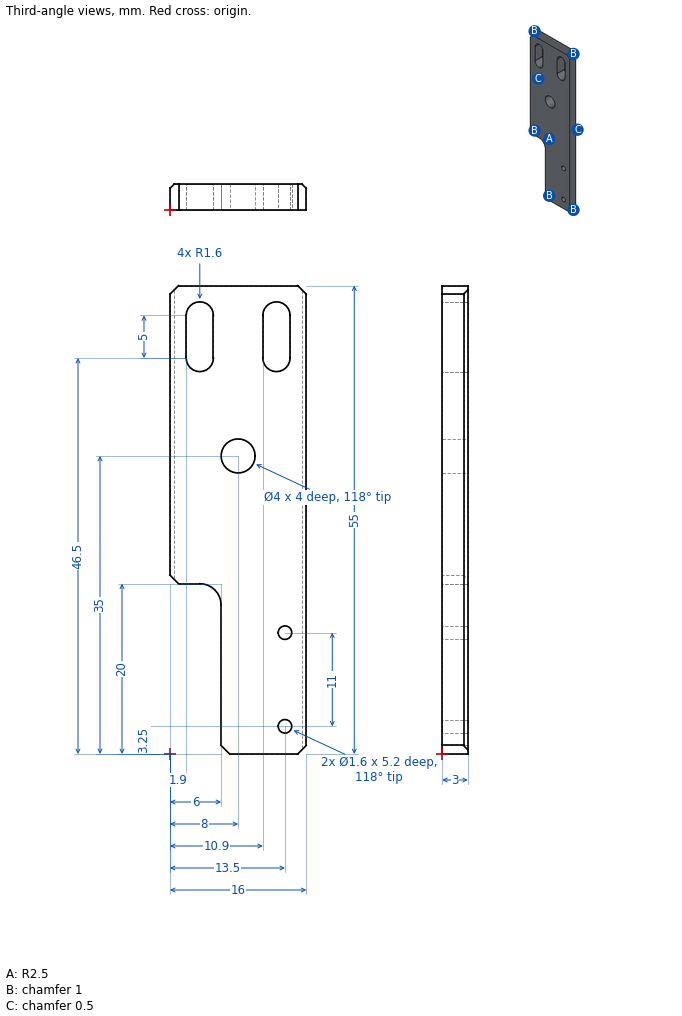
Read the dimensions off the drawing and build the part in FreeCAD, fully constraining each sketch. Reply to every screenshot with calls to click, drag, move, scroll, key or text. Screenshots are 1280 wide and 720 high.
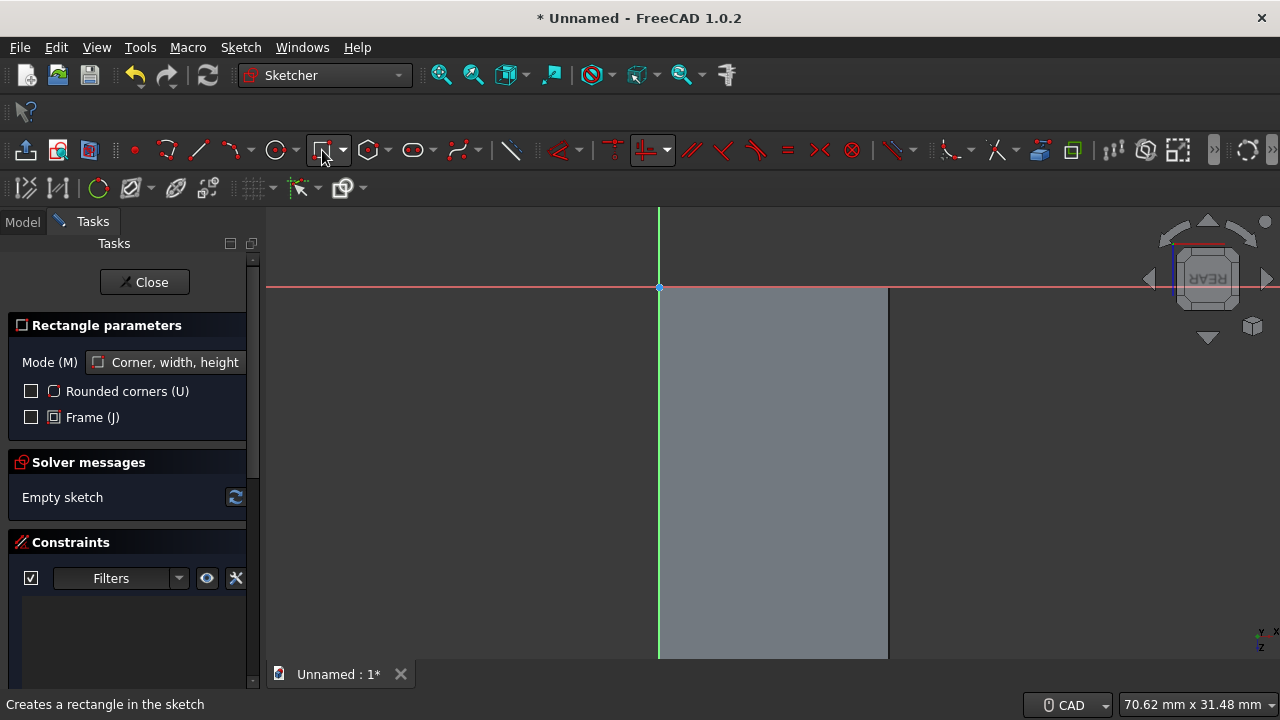
click(659, 287)
move(745, 574)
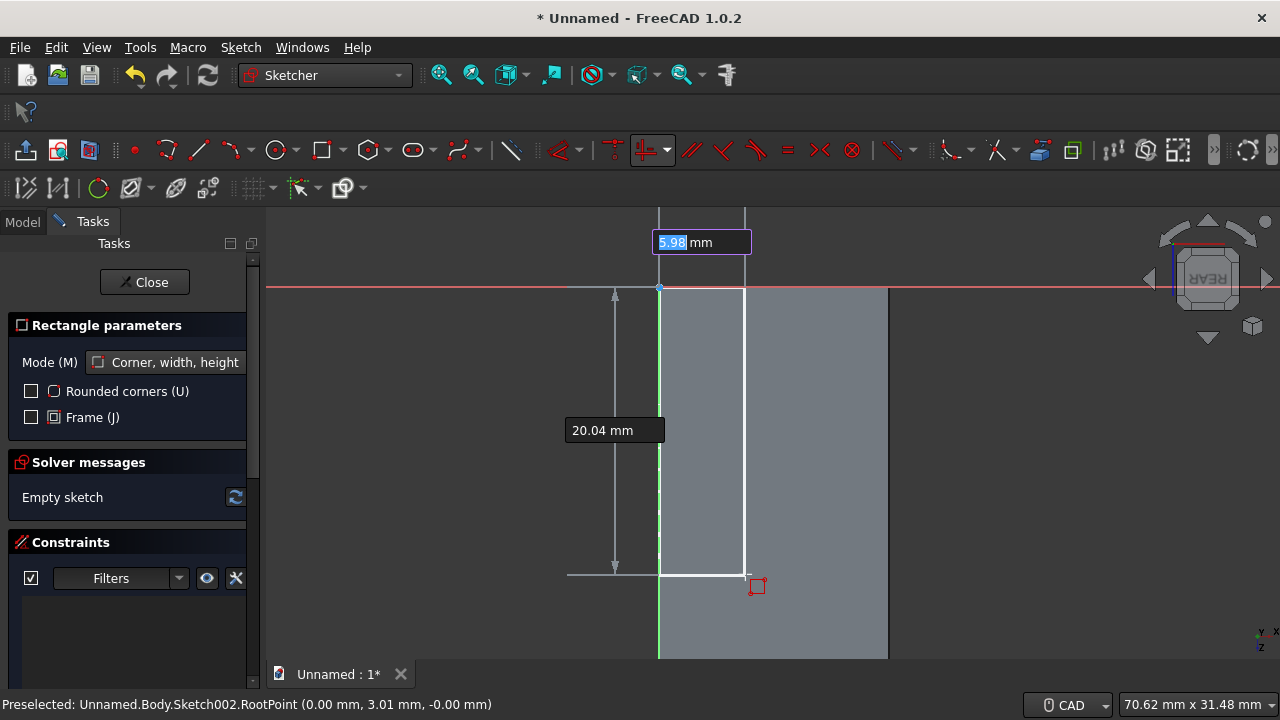
text(6)
key(Tab)
text(20)
key(Return)
key(Escape)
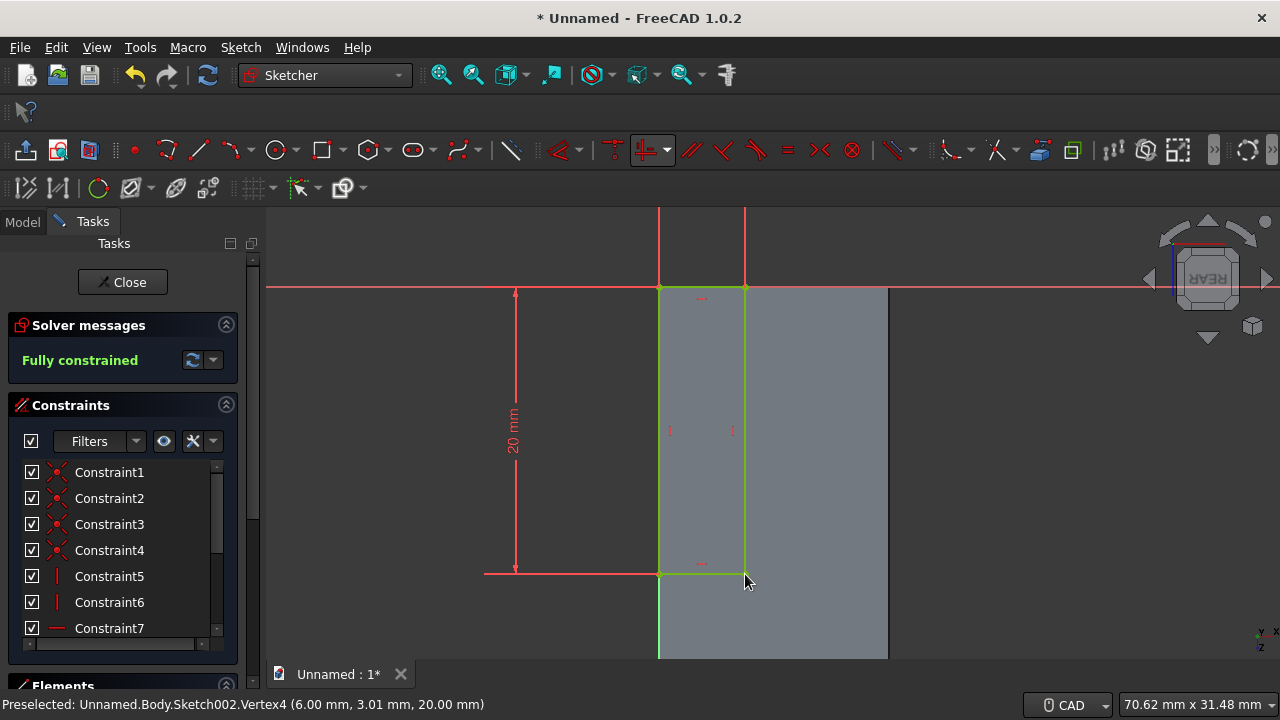
click(123, 282)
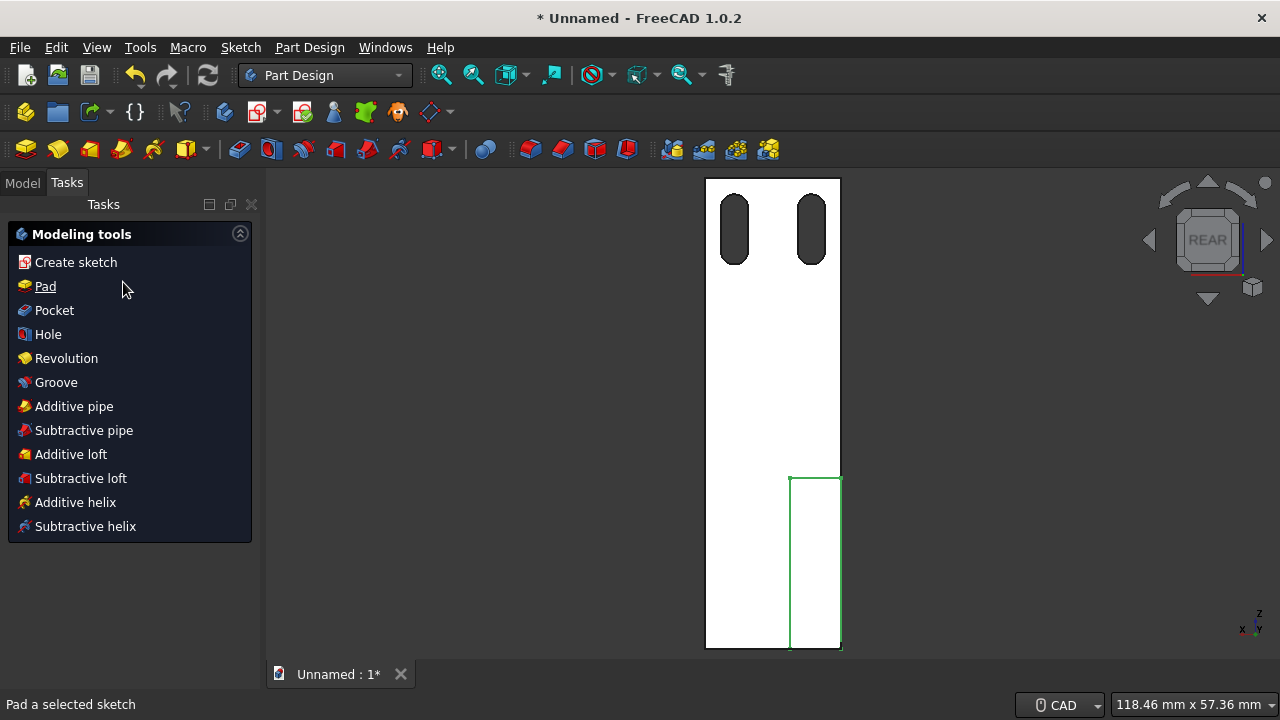
click(240, 150)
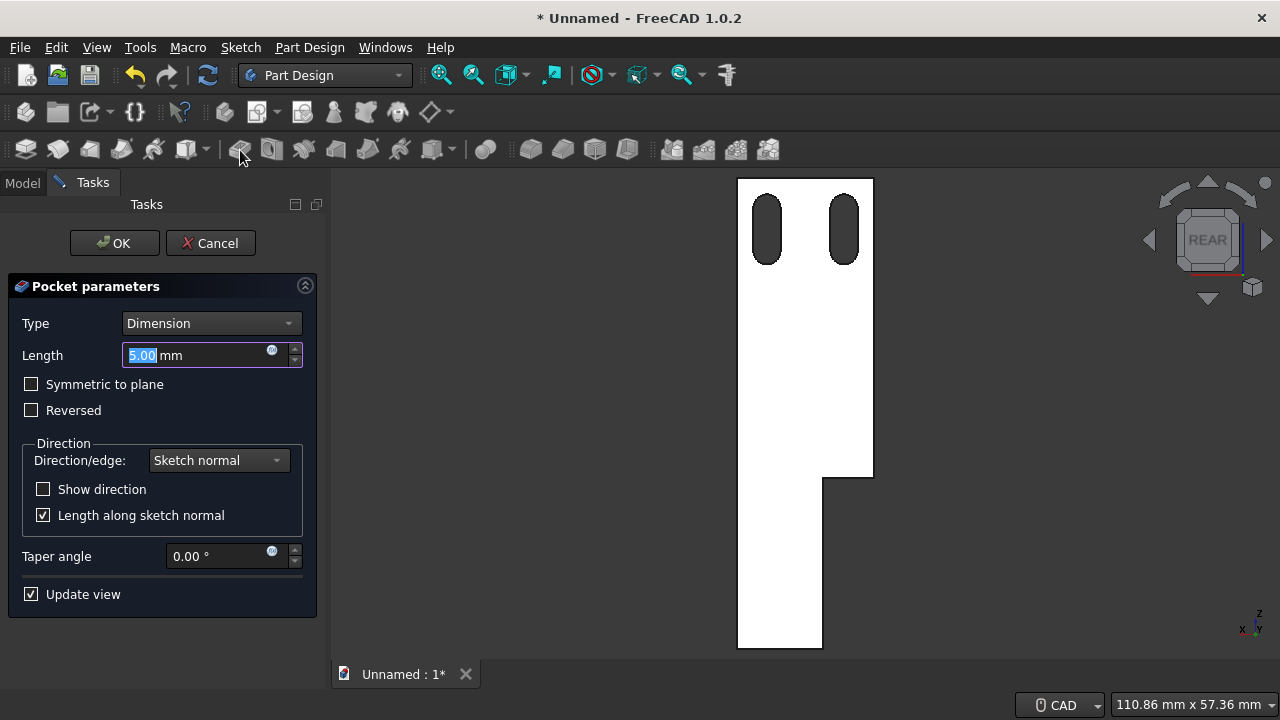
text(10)
key(Tab)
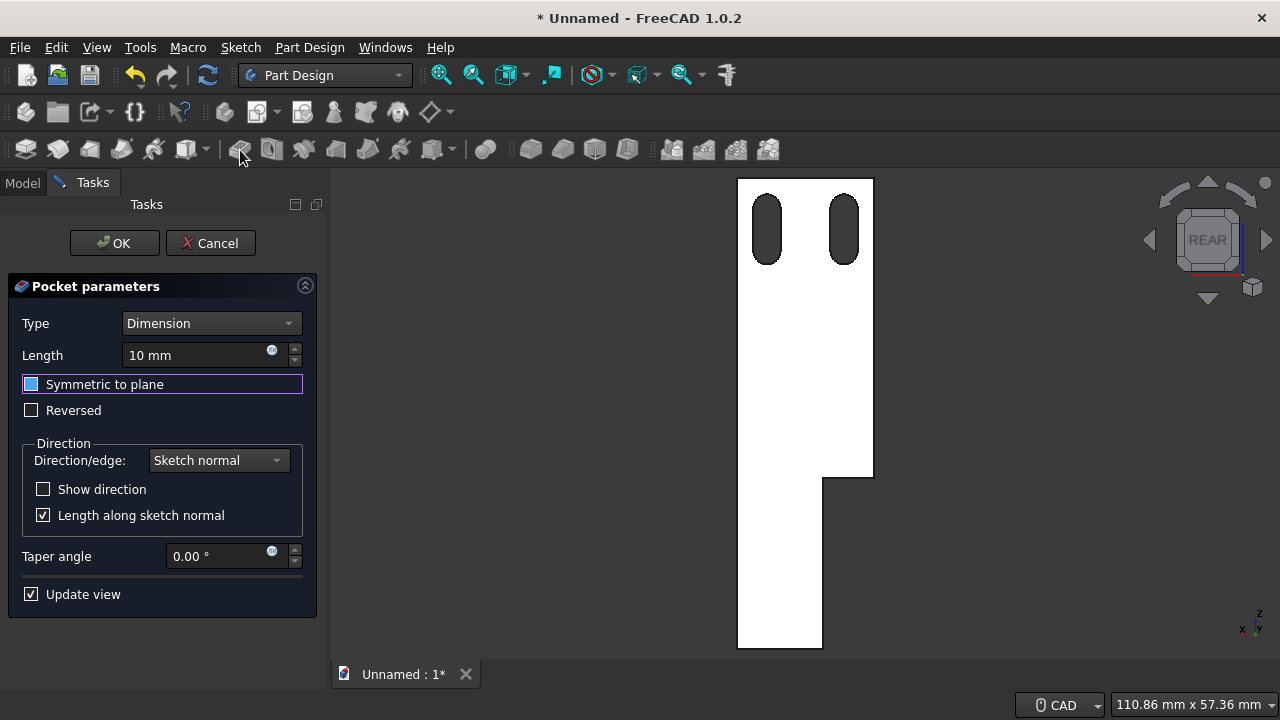
click(115, 243)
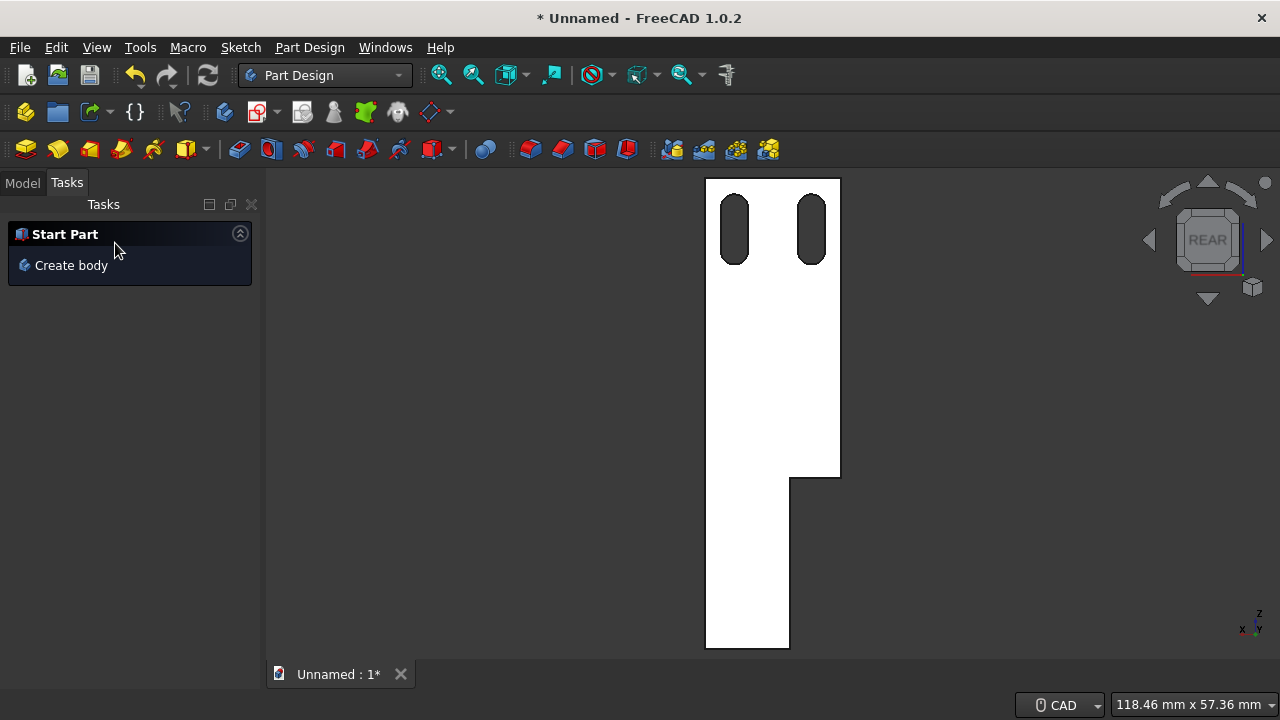
key(0)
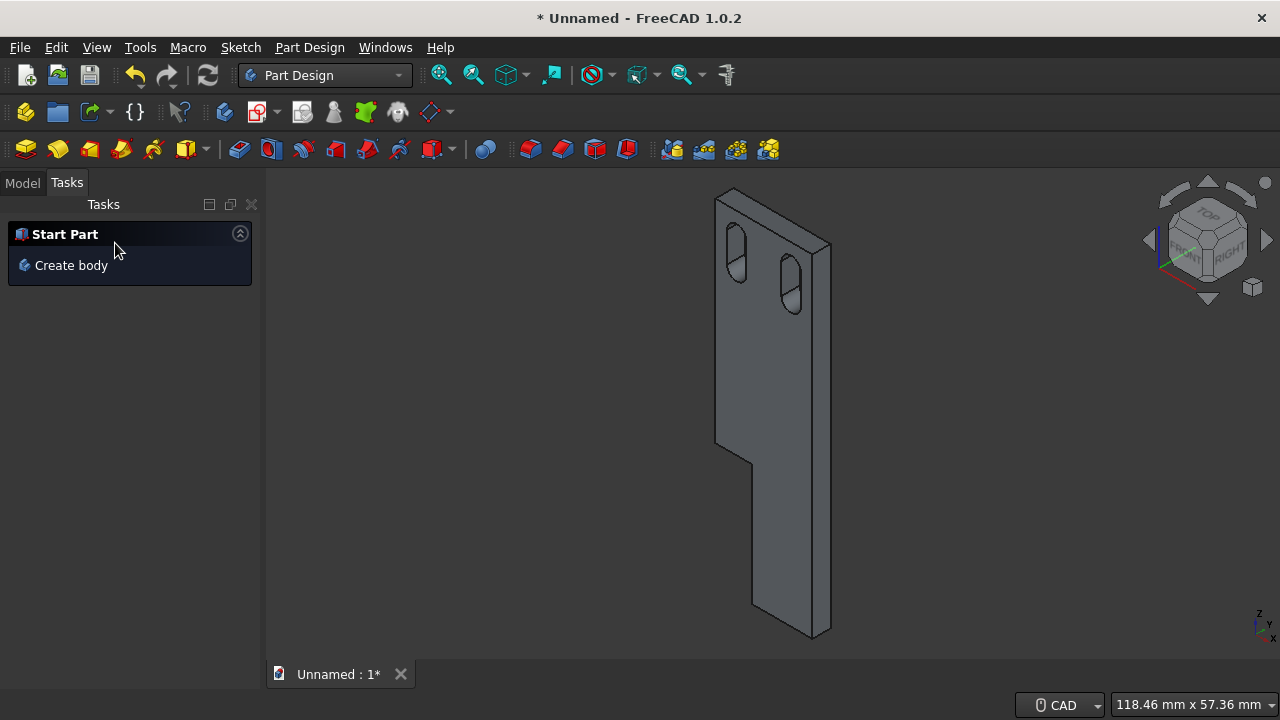
key(2)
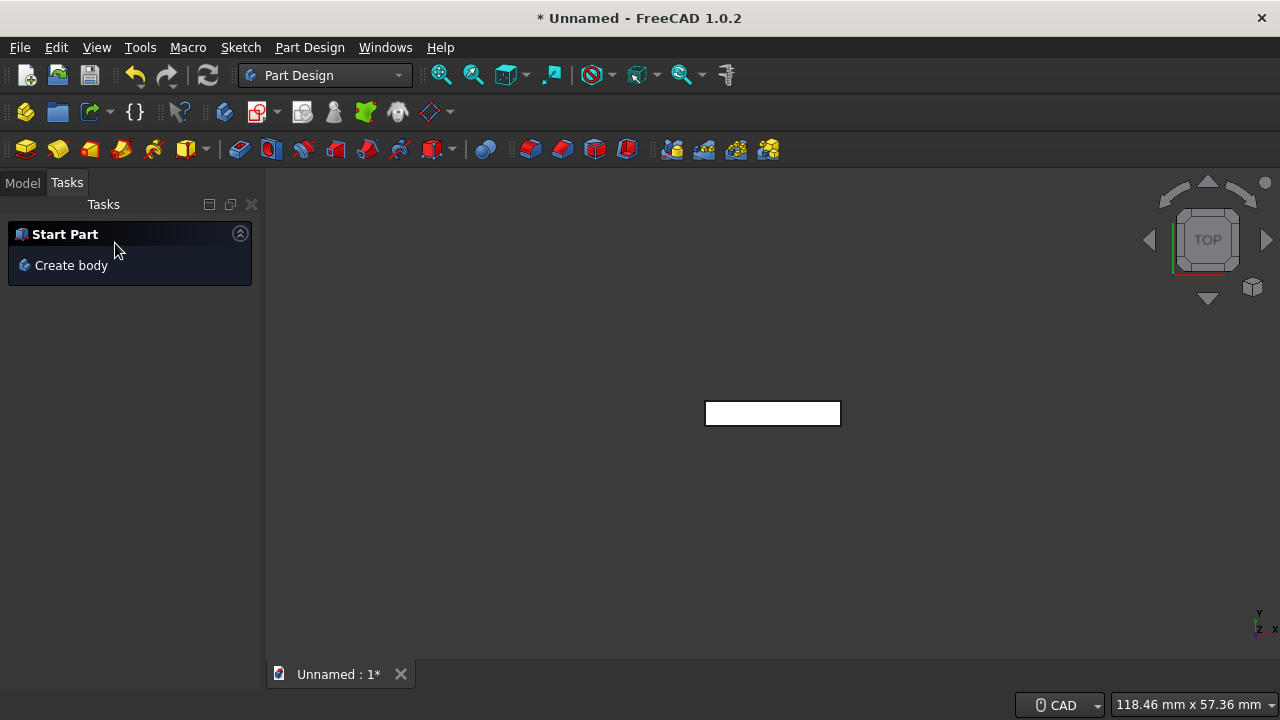
click(442, 76)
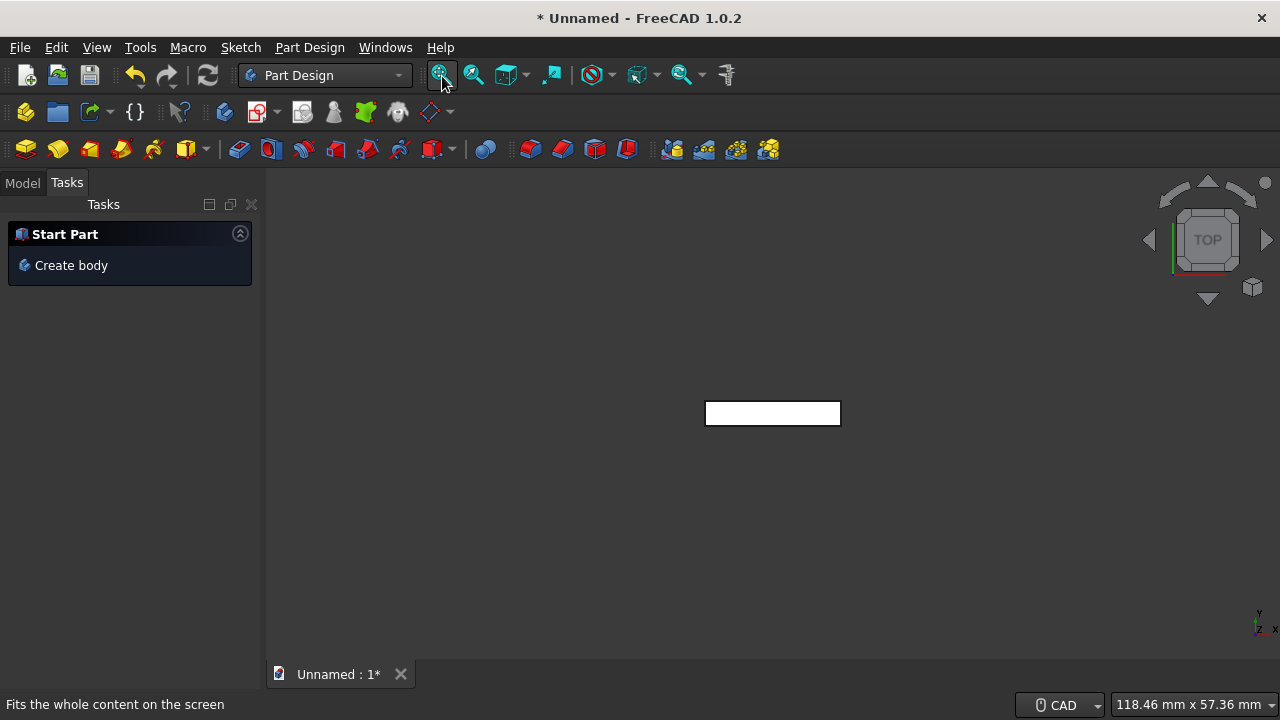
key(1)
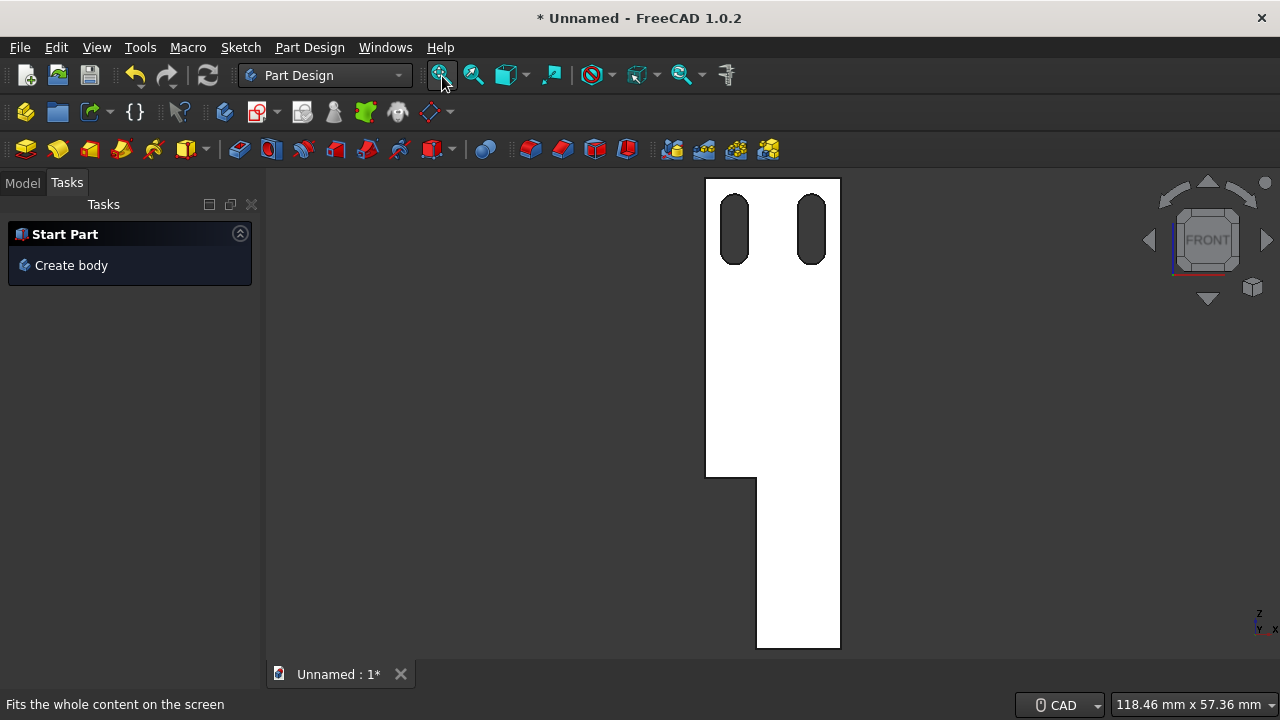
key(3)